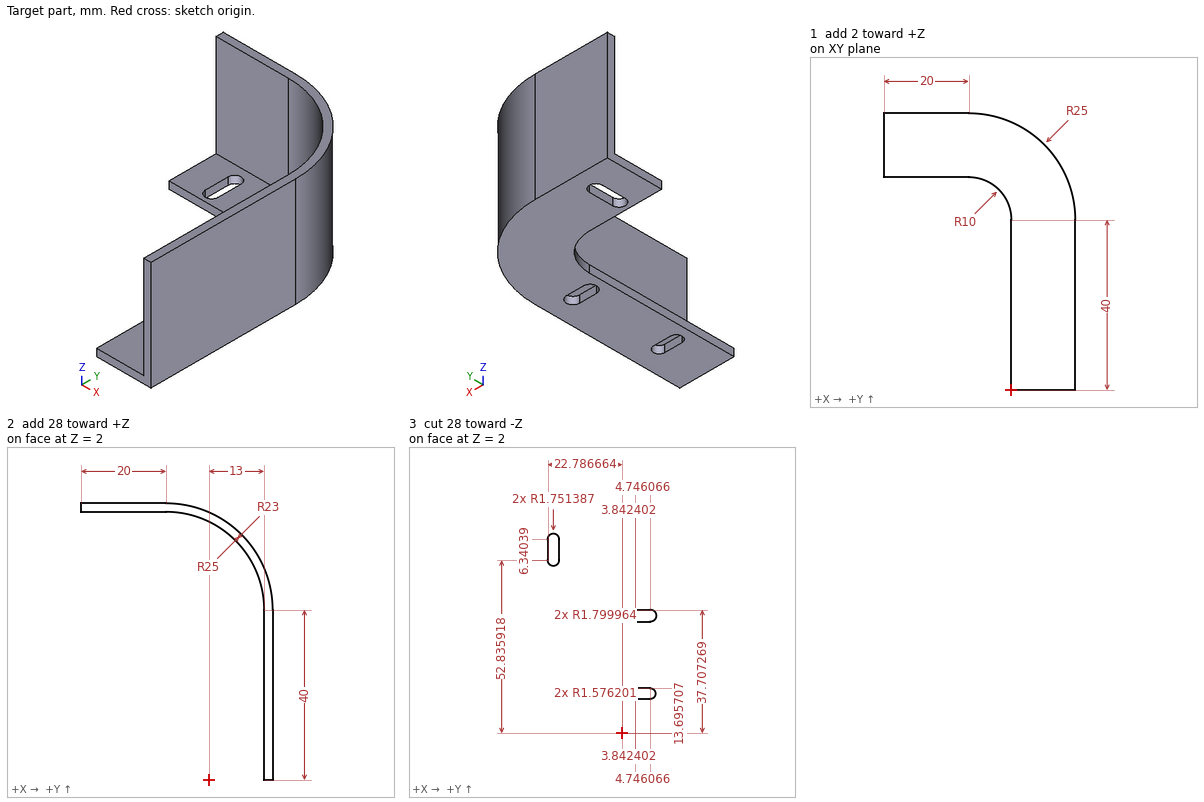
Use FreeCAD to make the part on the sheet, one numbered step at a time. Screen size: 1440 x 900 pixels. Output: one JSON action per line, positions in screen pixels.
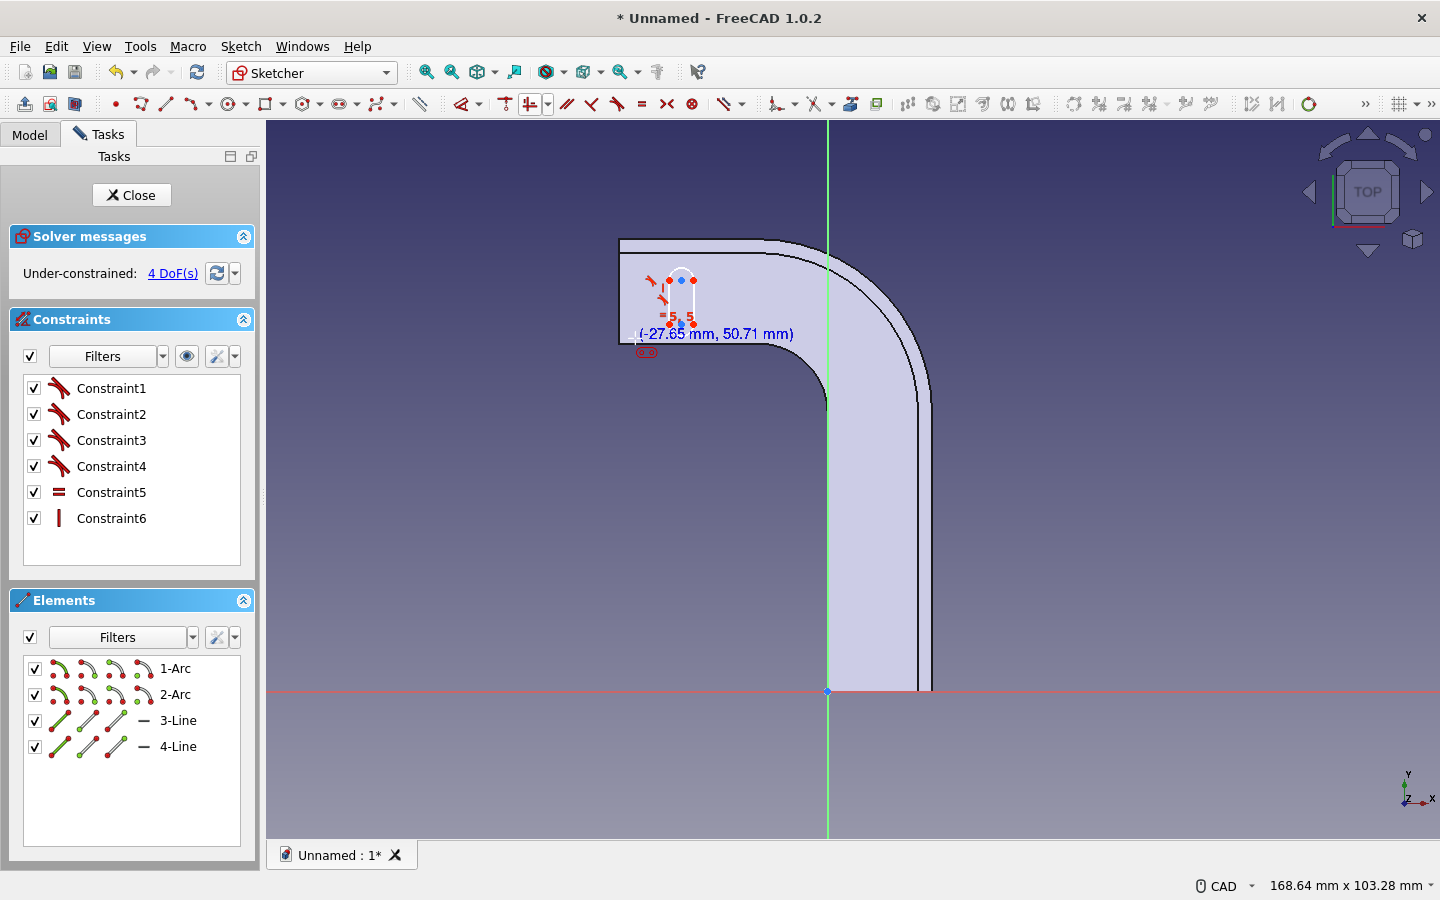
{"action": "scroll", "coordinate": [854, 607], "scroll_direction": "up", "scroll_amount": 4}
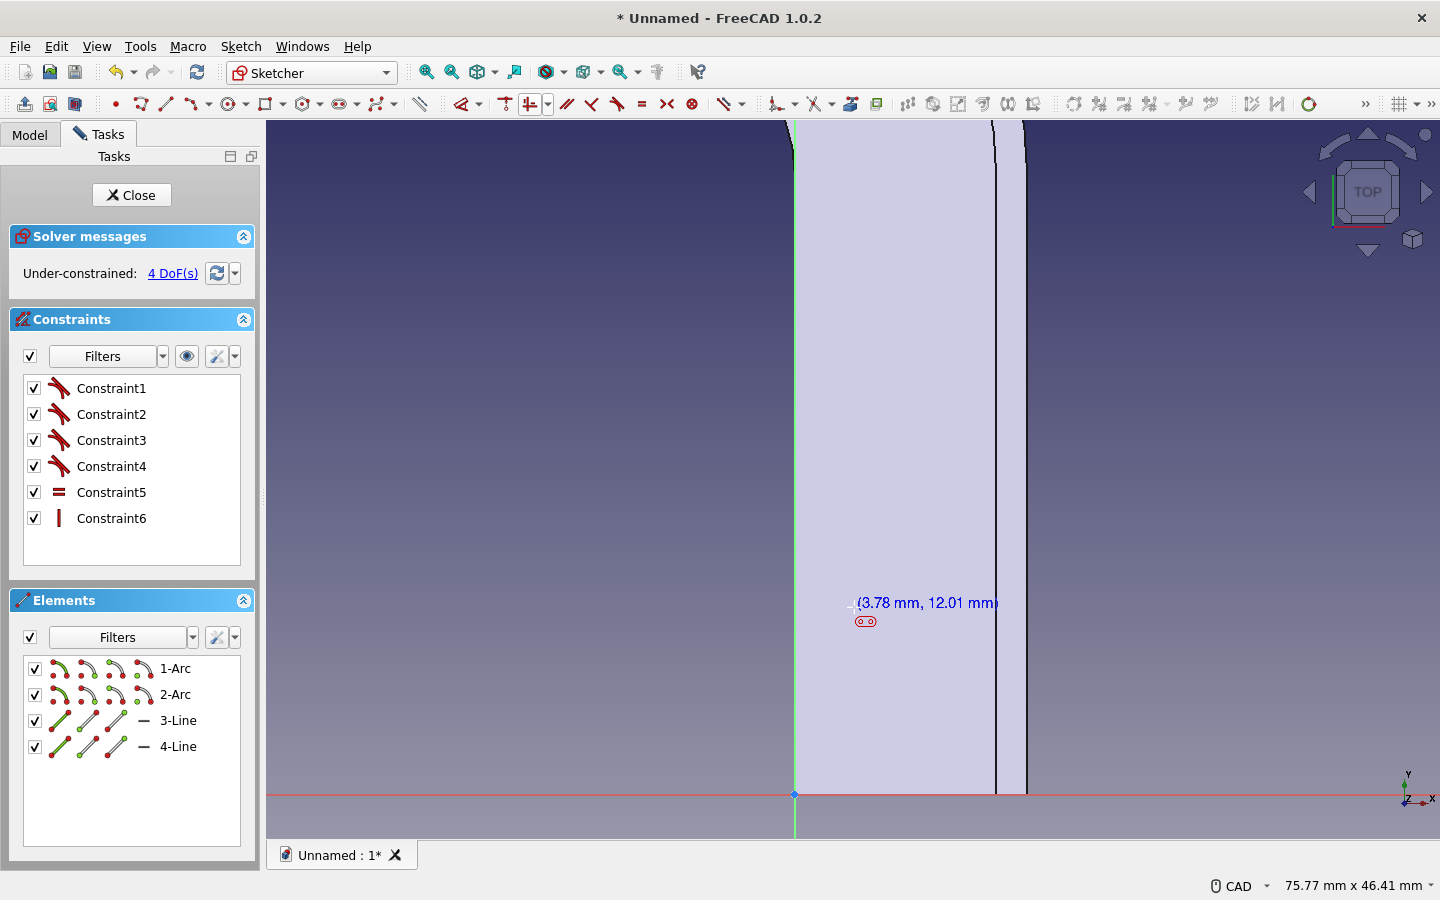
{"action": "left_click", "coordinate": [854, 607]}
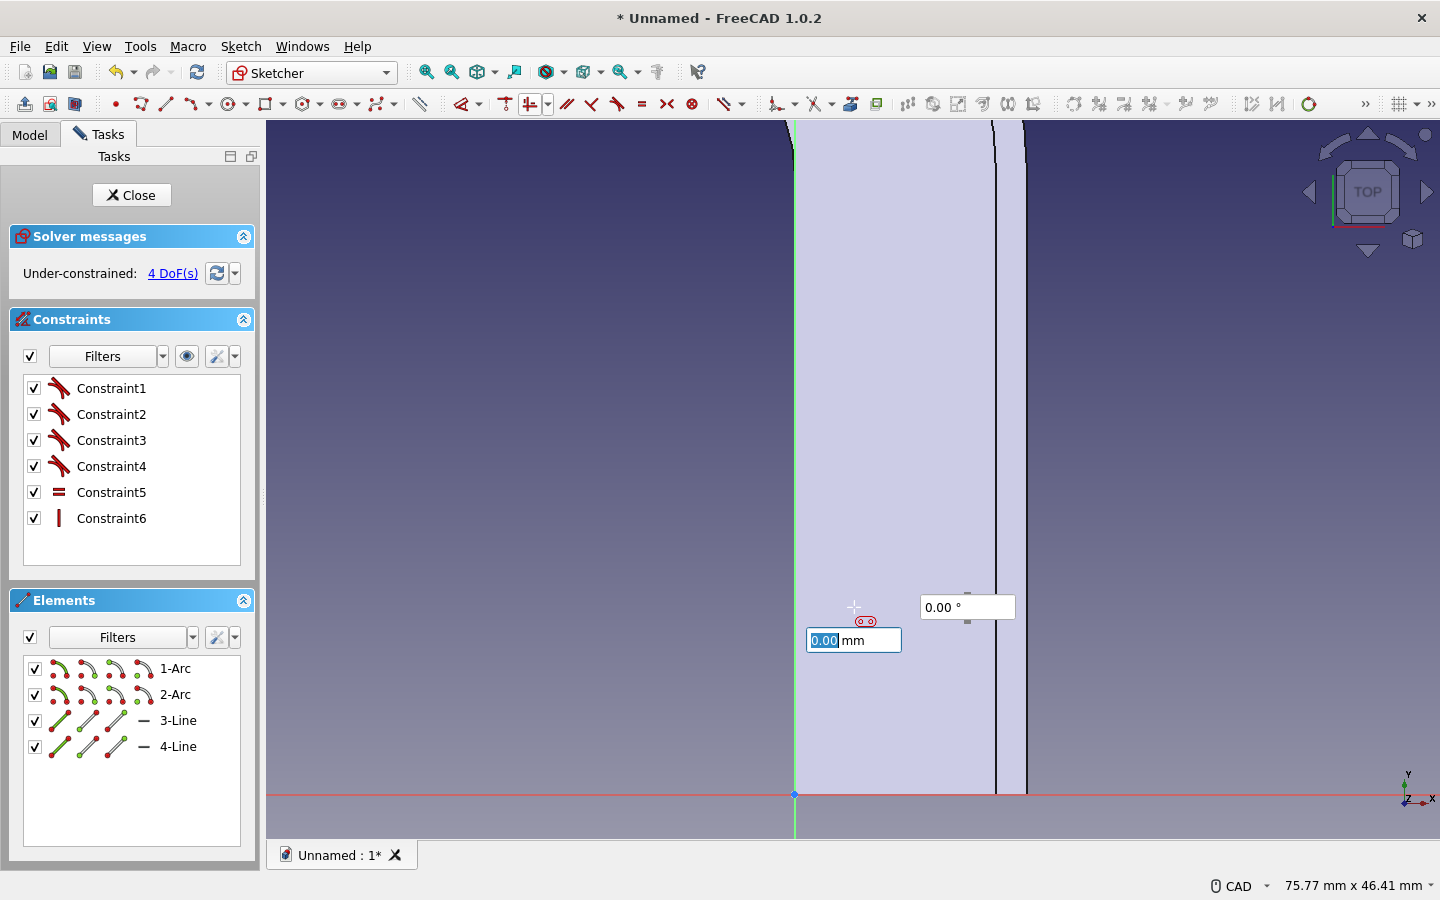
{"action": "left_click", "coordinate": [928, 607]}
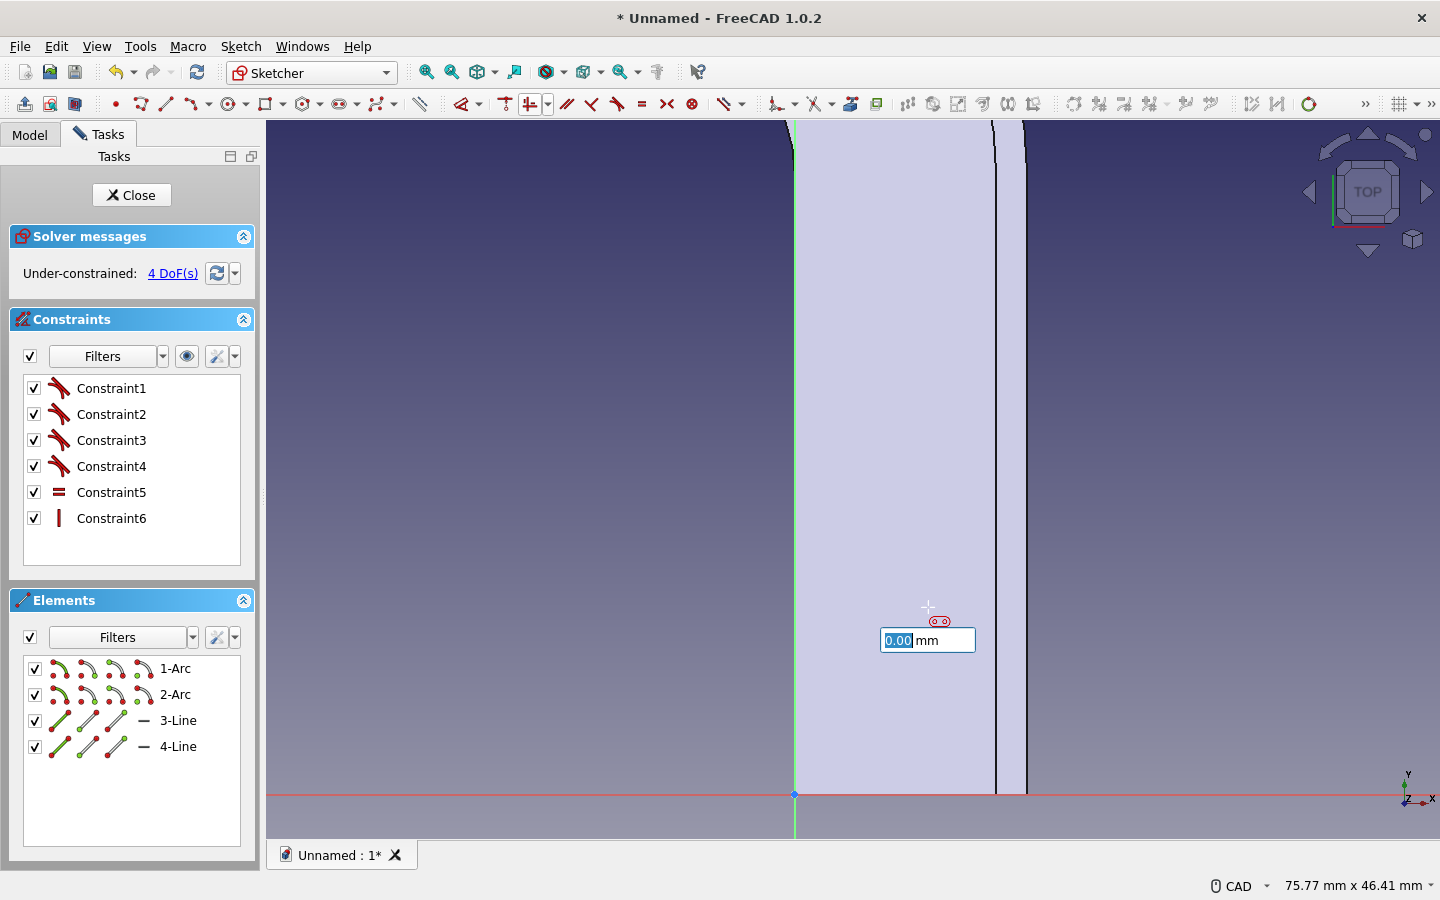
{"action": "left_click", "coordinate": [891, 582]}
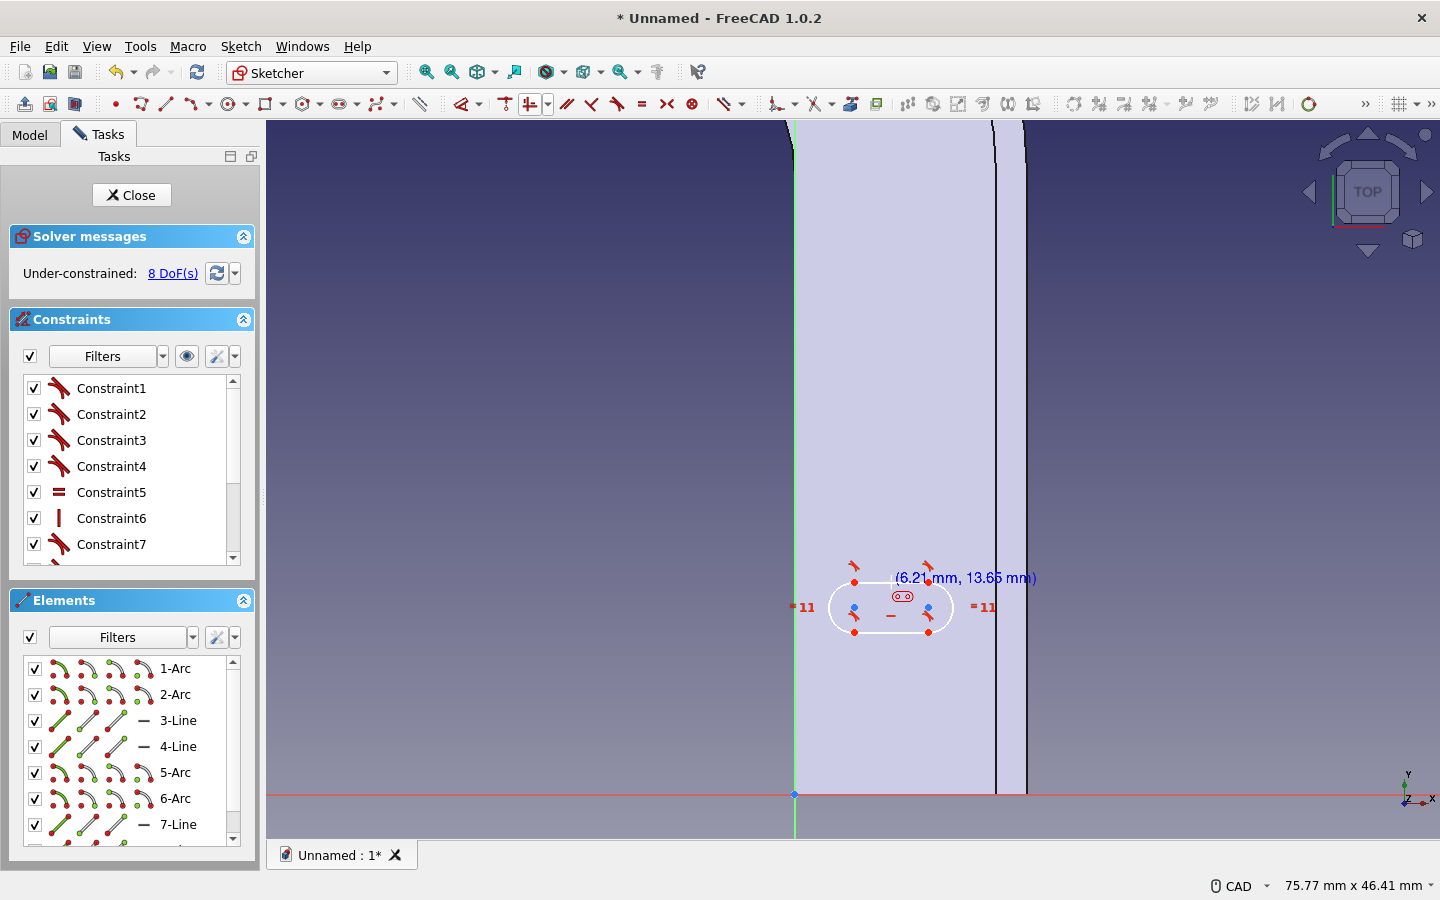
{"action": "left_click", "coordinate": [854, 238]}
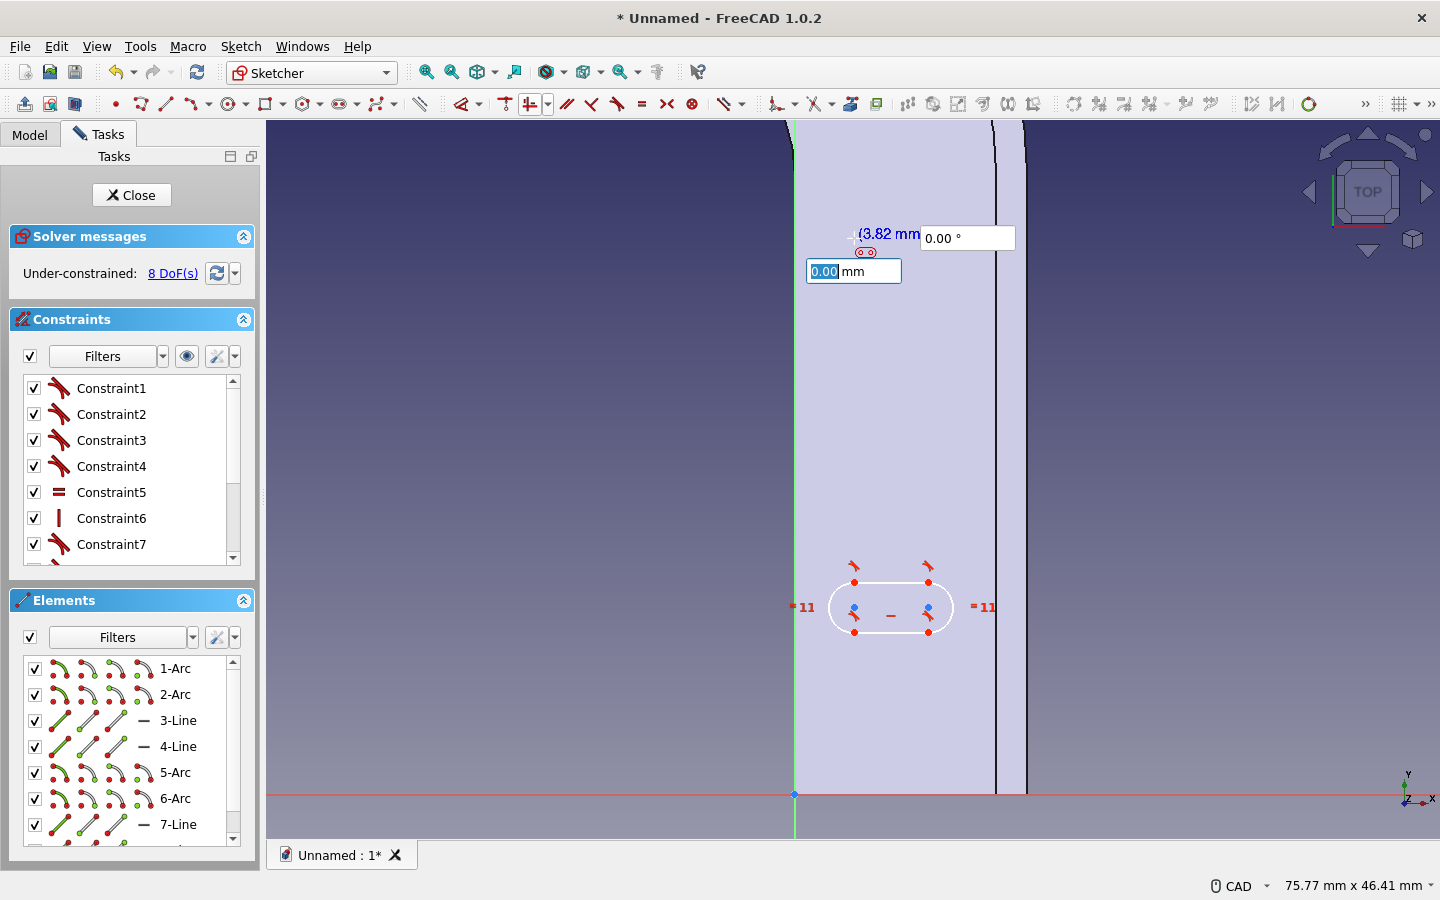
{"action": "left_click", "coordinate": [928, 238]}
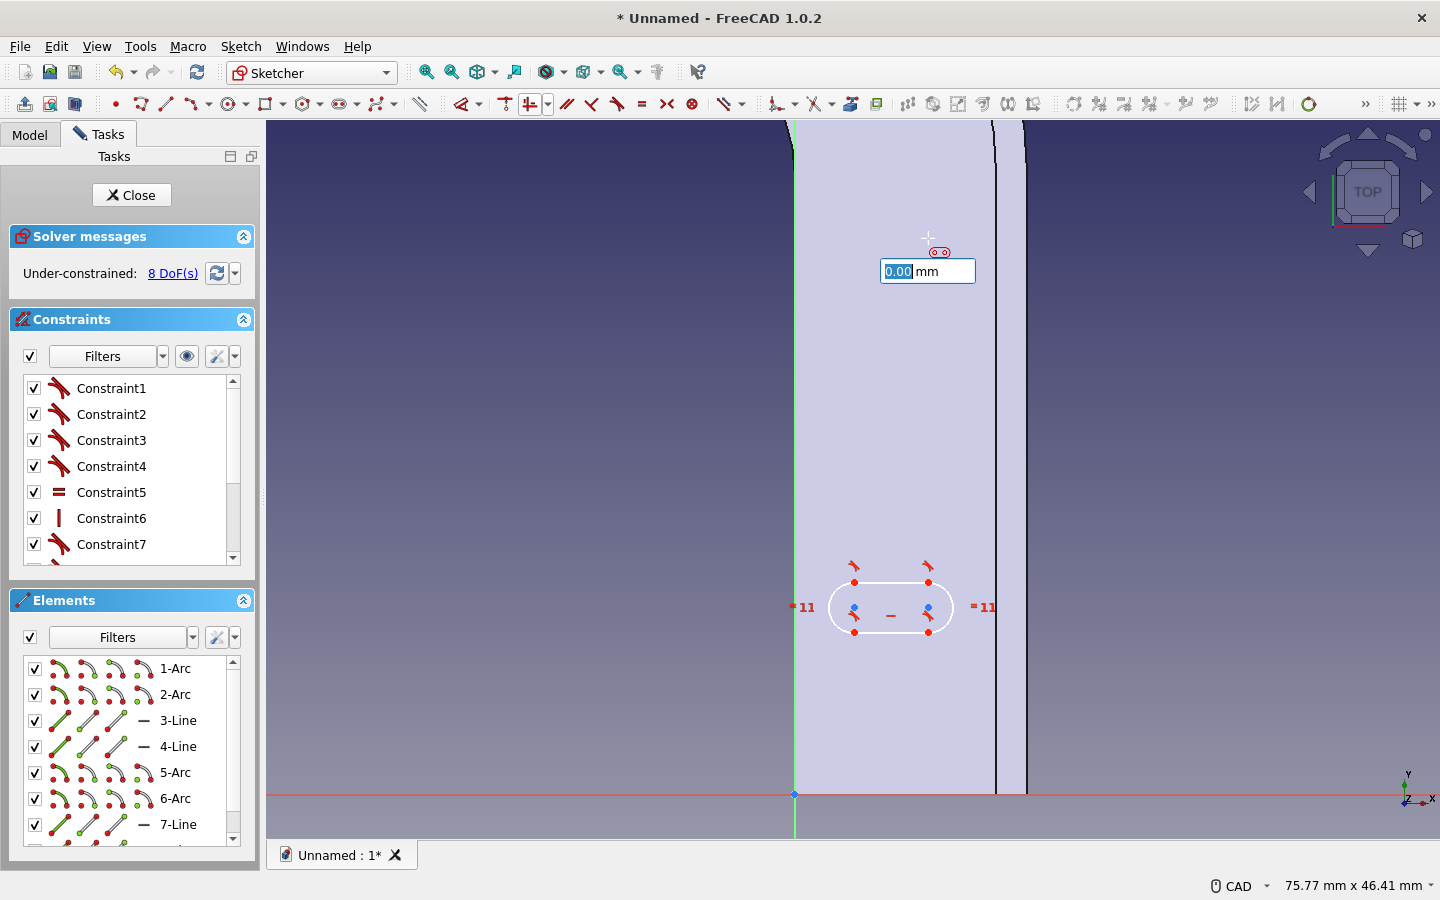
{"action": "left_click", "coordinate": [891, 210]}
{"action": "key", "text": "Escape"}